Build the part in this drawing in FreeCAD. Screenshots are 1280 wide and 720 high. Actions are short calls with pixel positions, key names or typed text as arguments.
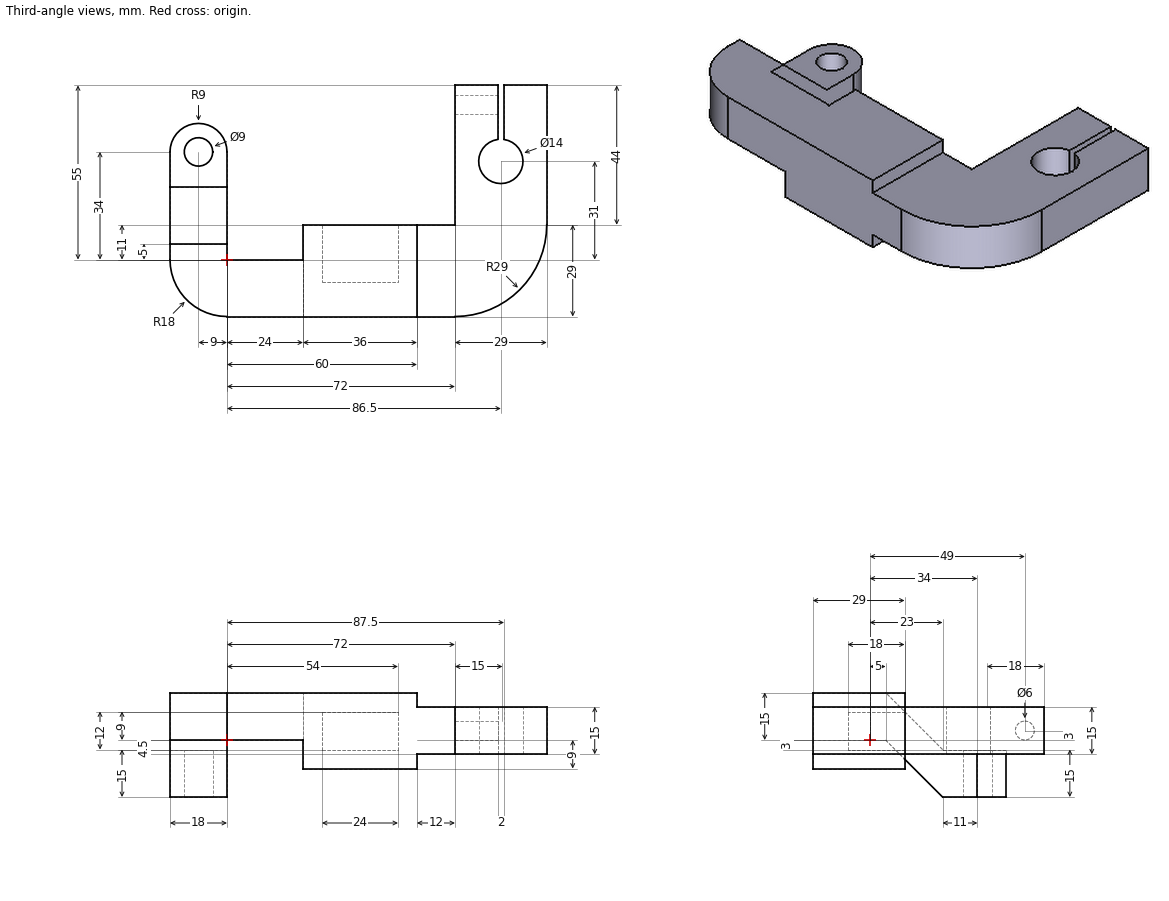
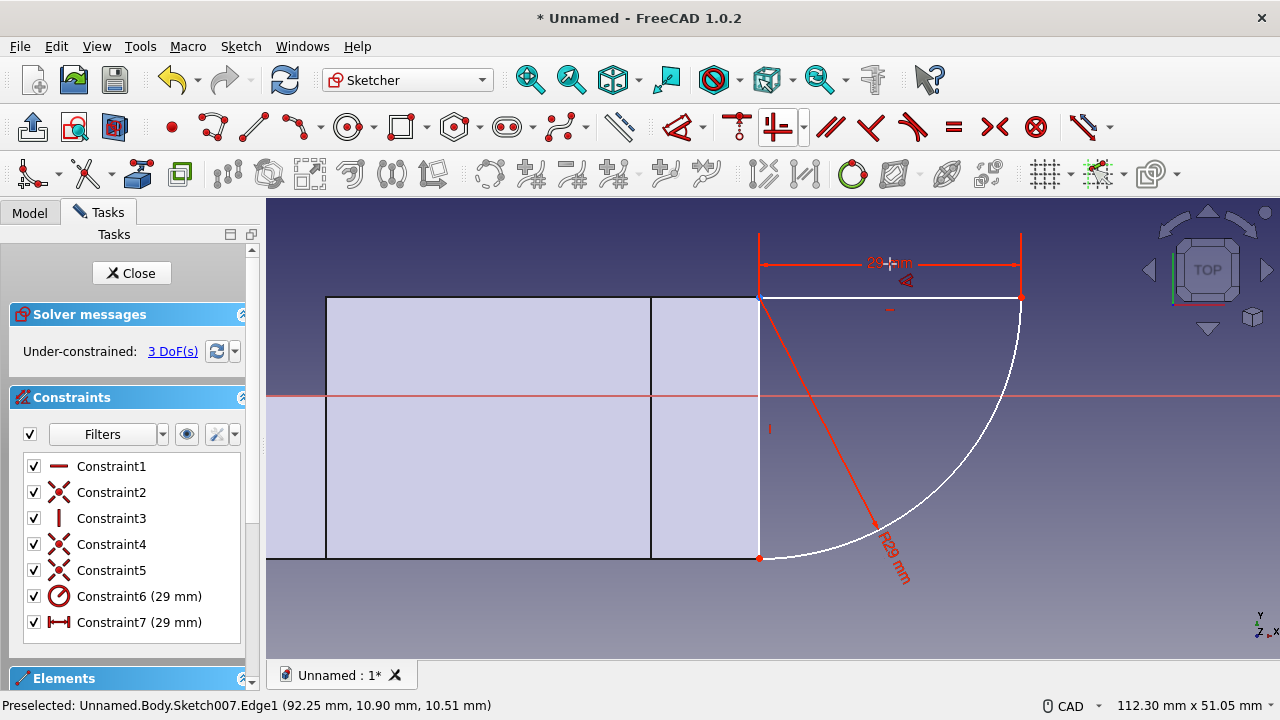
click(759, 376)
click(725, 428)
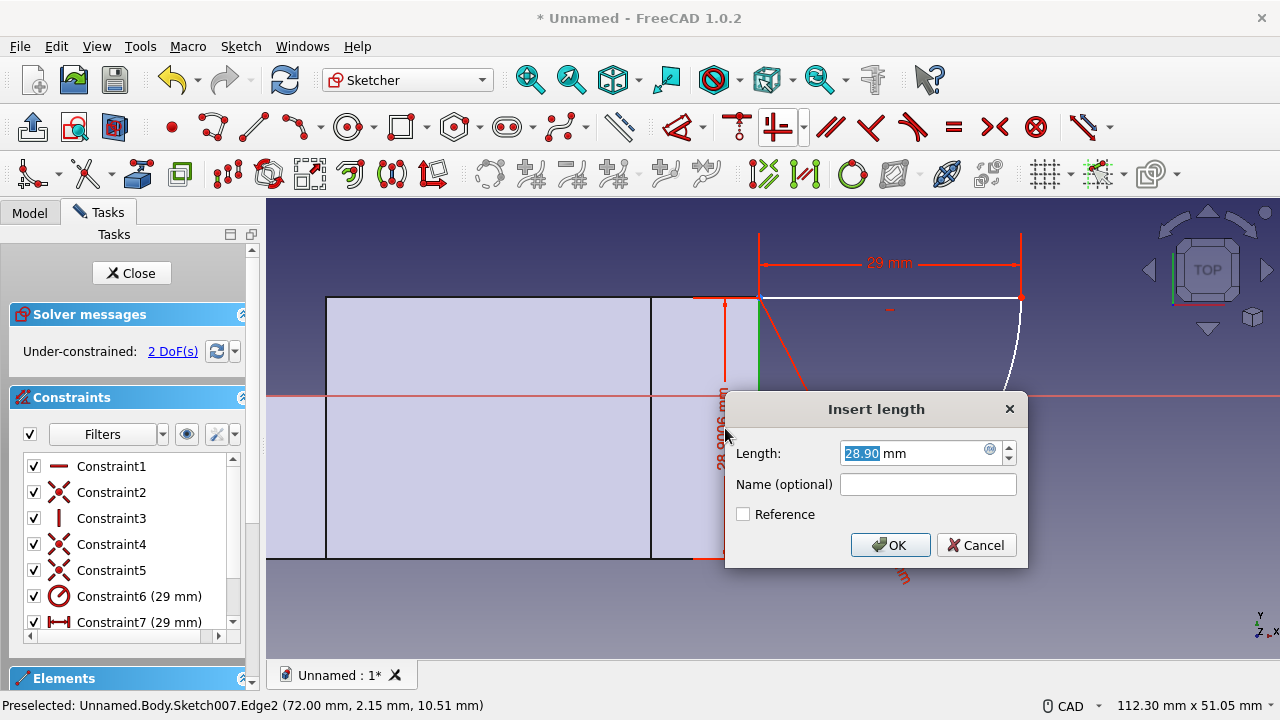
text(29)
key(Return)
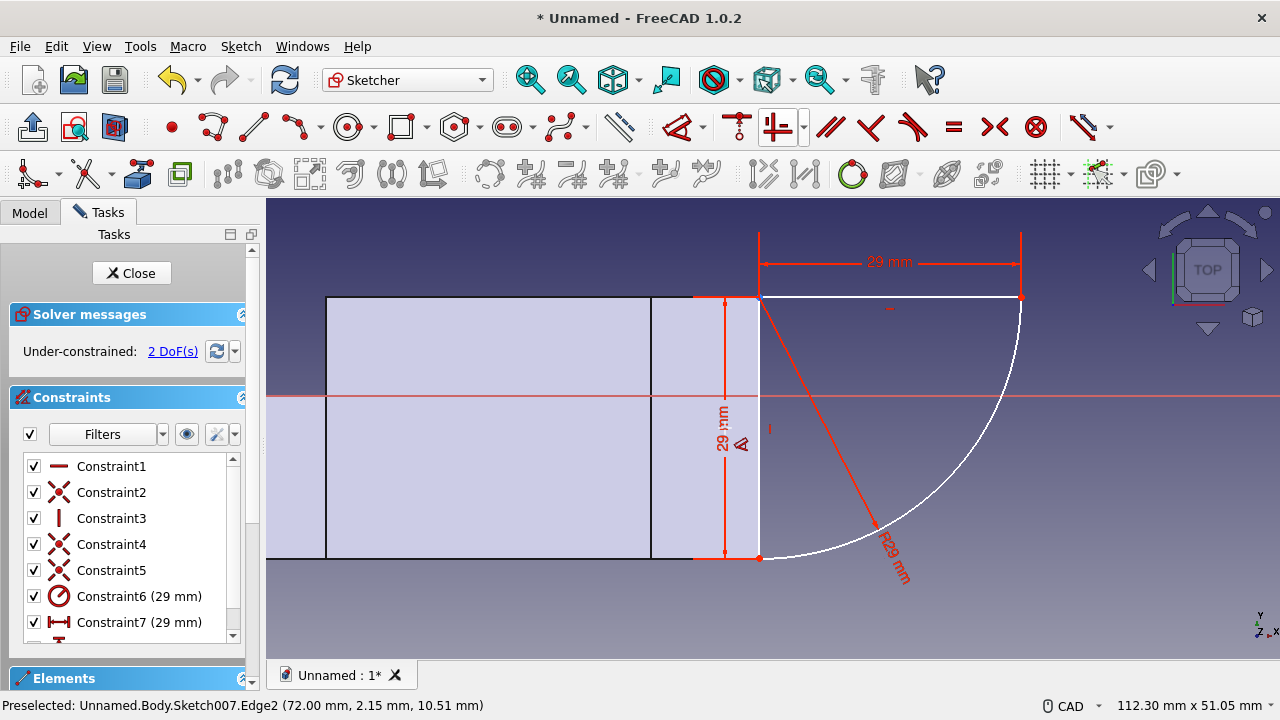
click(1021, 297)
click(1055, 347)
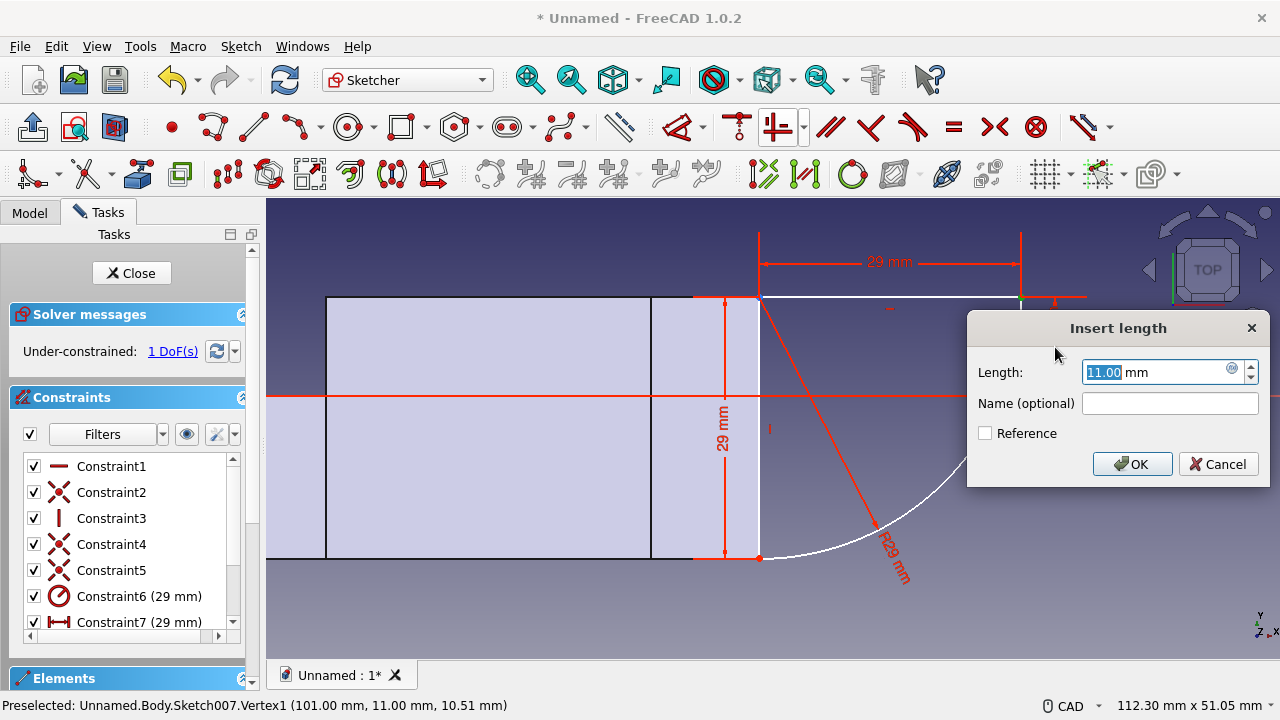
text(11)
key(Return)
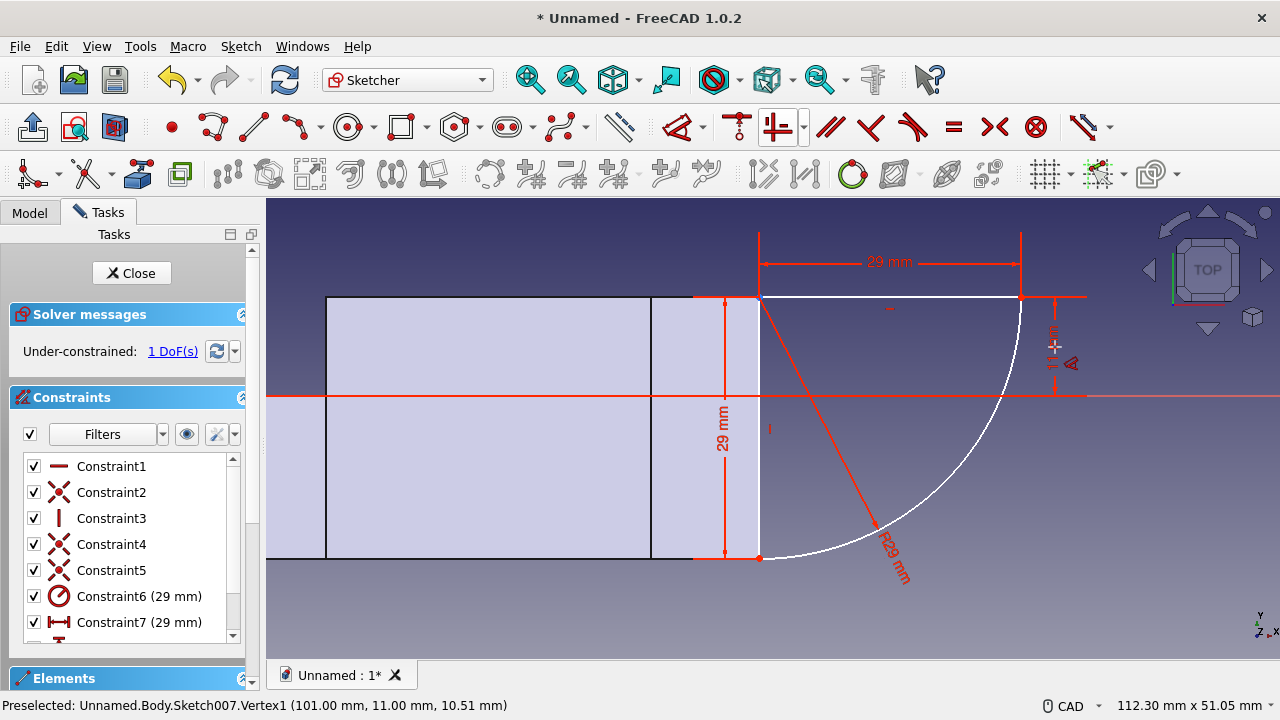
click(759, 297)
click(527, 263)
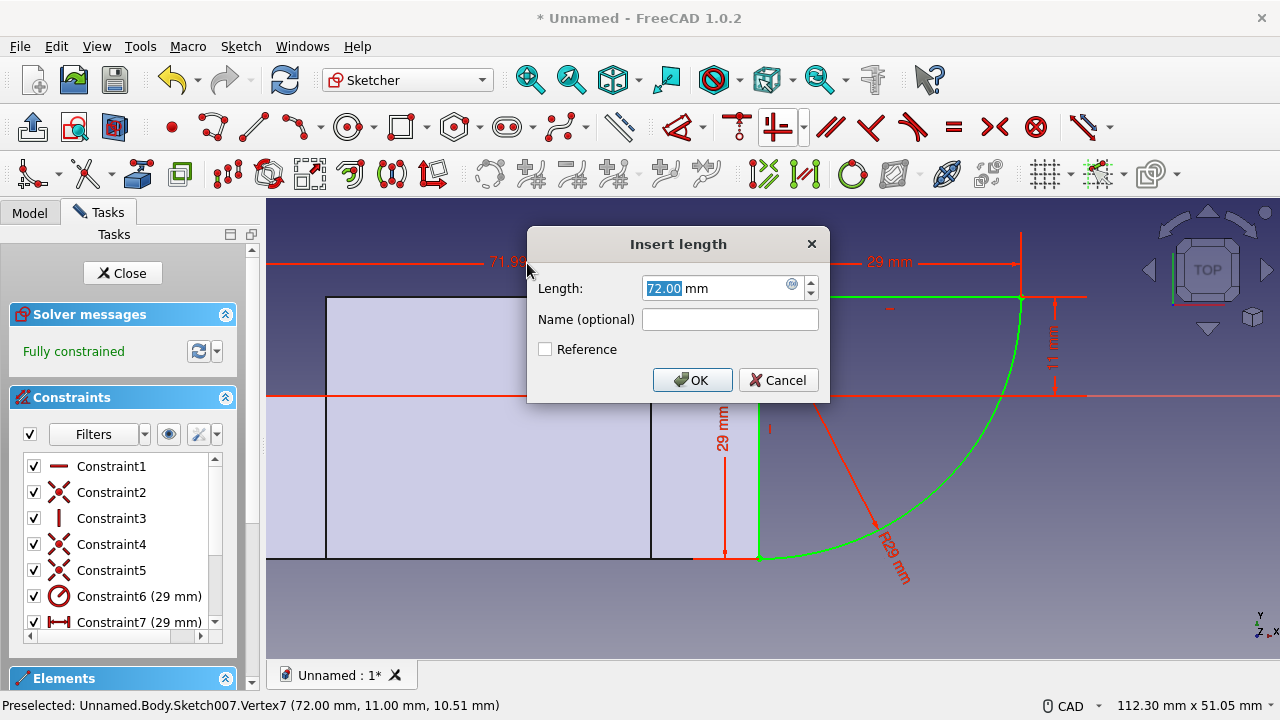
text(72)
key(Return)
key(Escape)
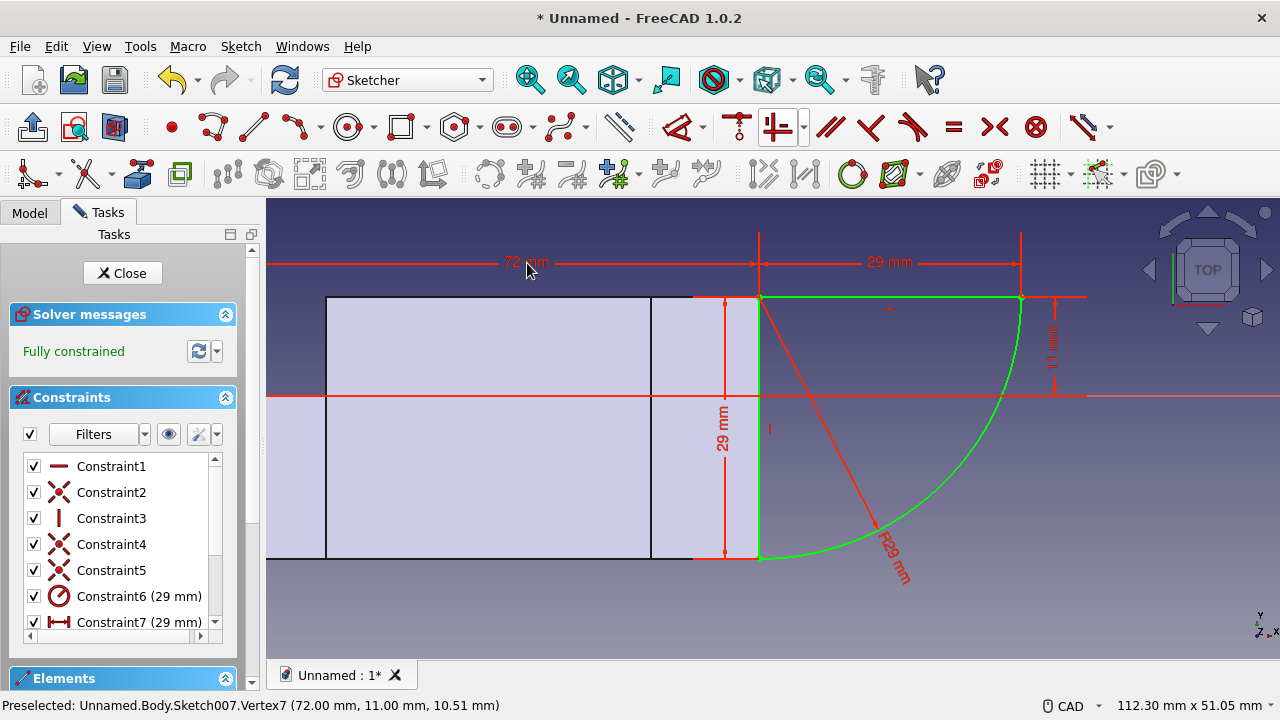
click(123, 273)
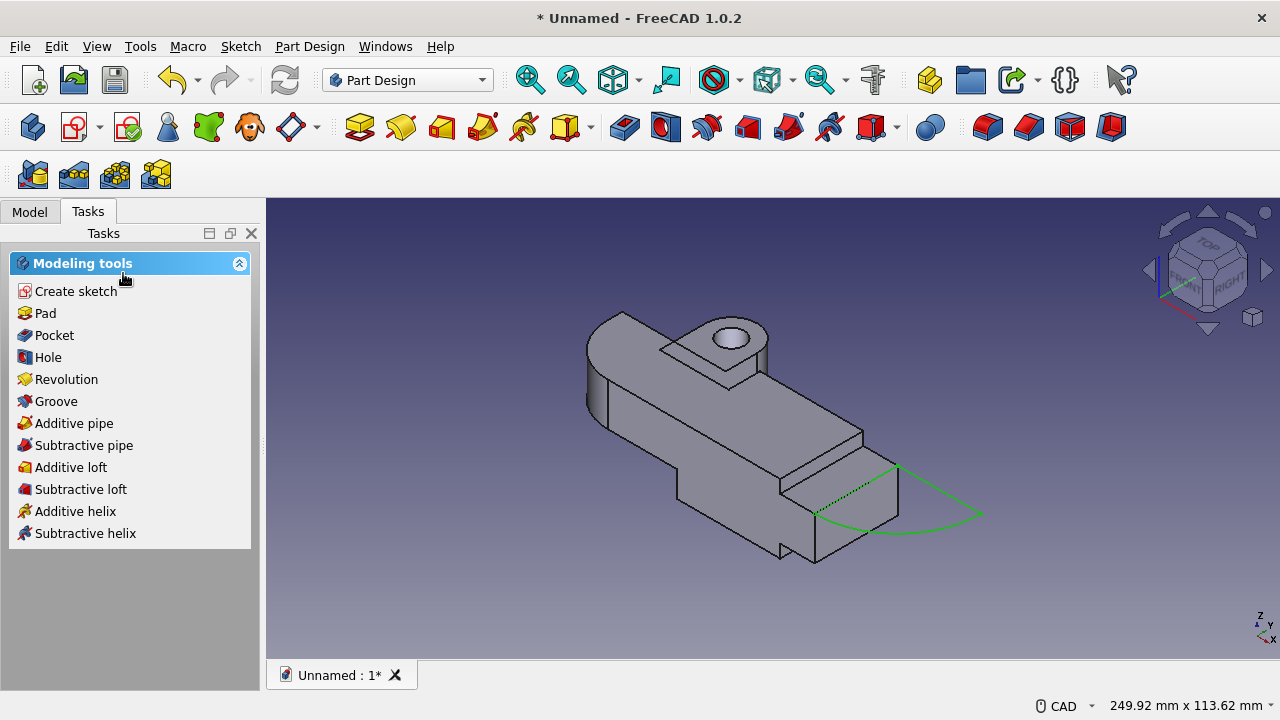
click(360, 128)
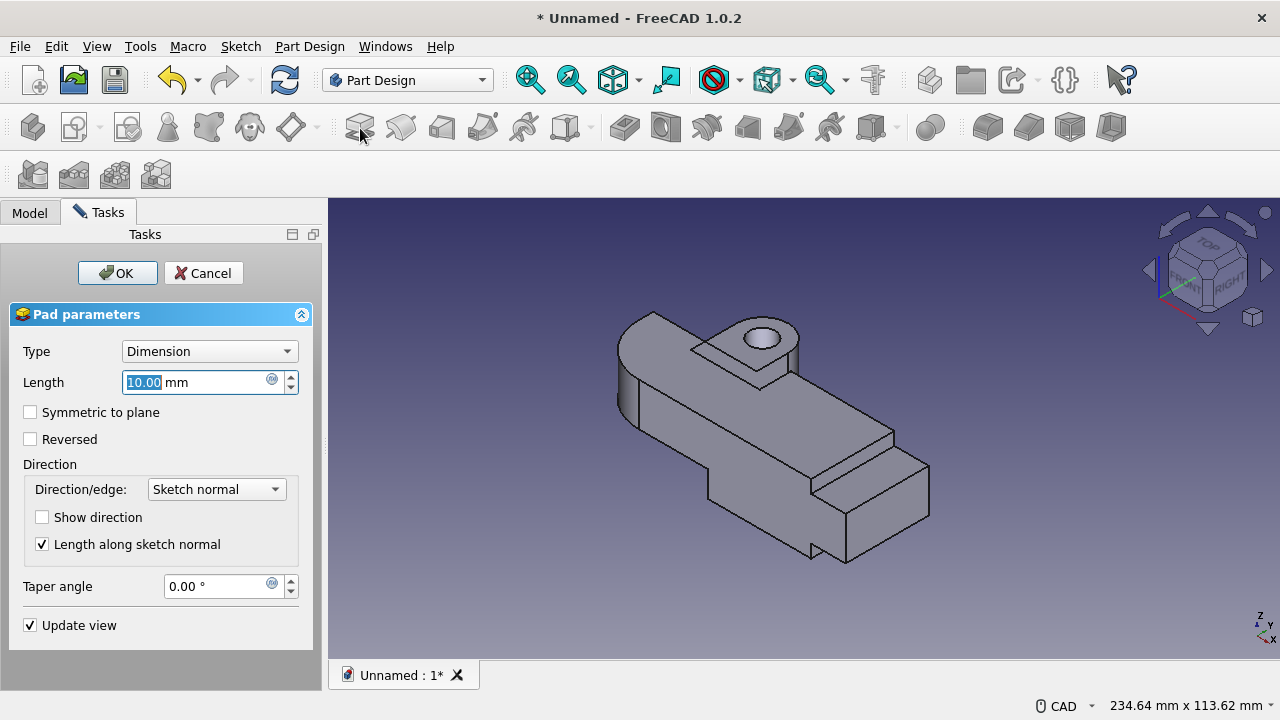
text(15)
key(Tab)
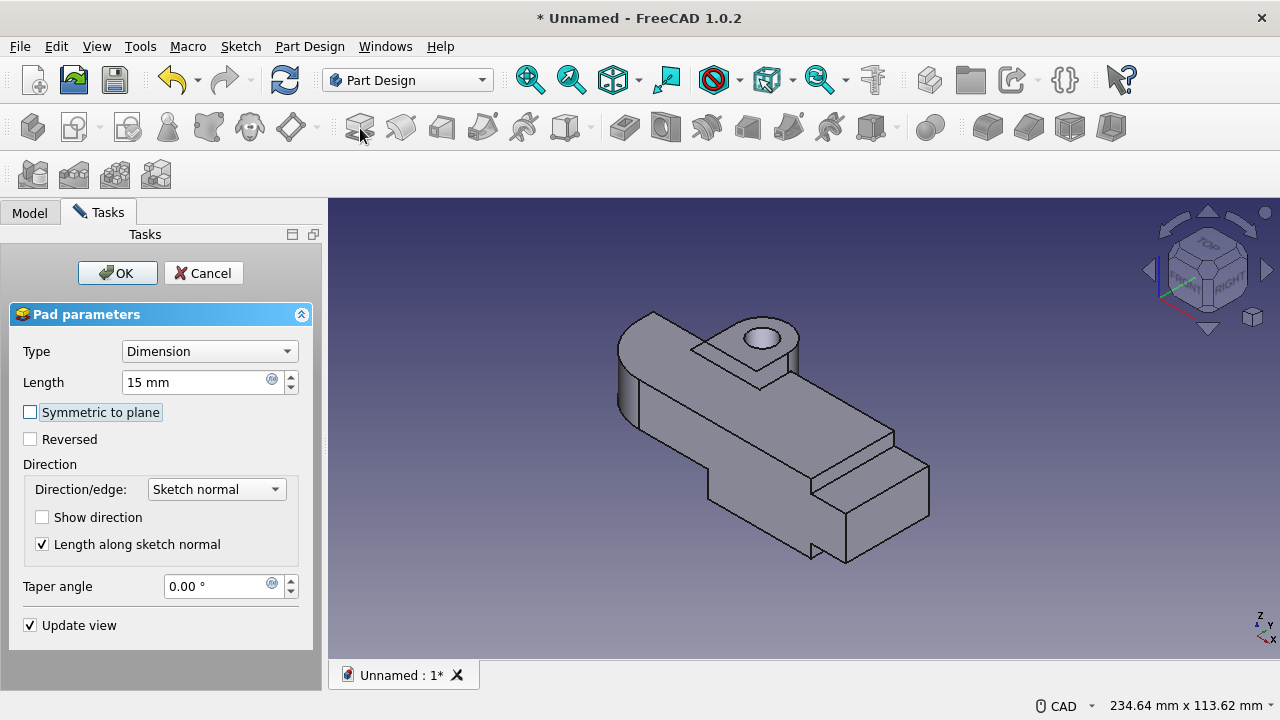
click(31, 439)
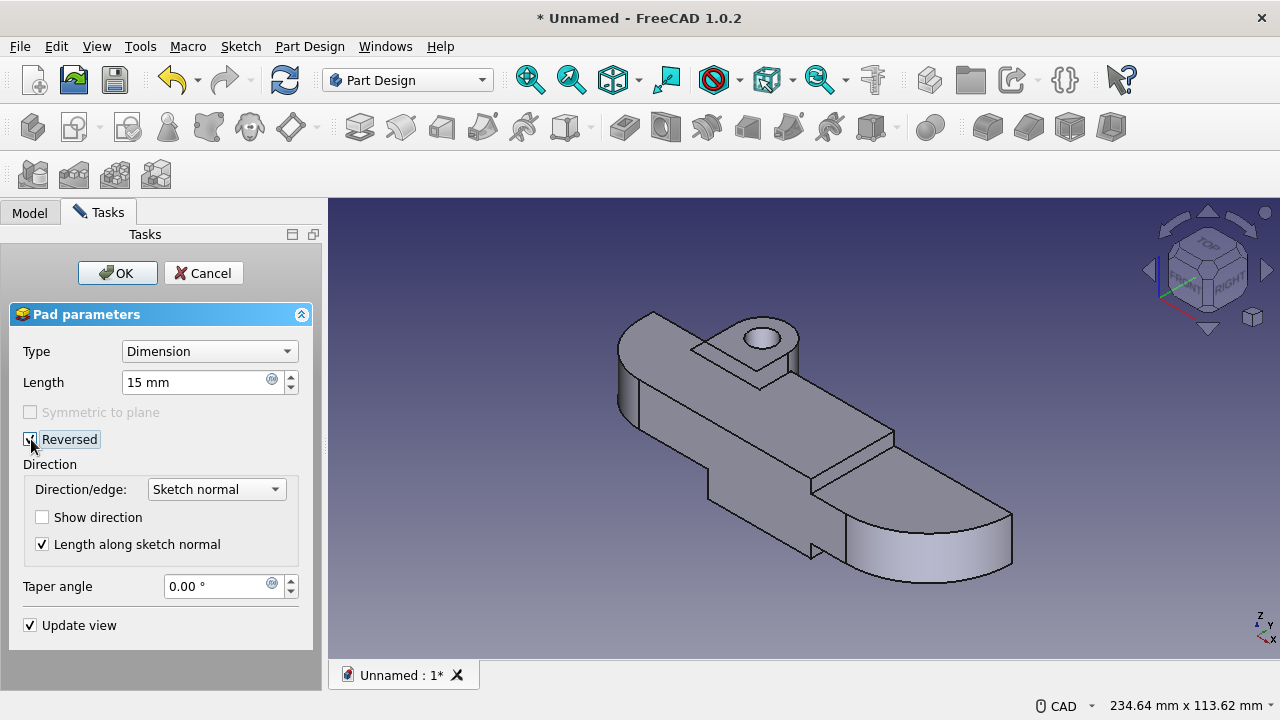
click(118, 273)